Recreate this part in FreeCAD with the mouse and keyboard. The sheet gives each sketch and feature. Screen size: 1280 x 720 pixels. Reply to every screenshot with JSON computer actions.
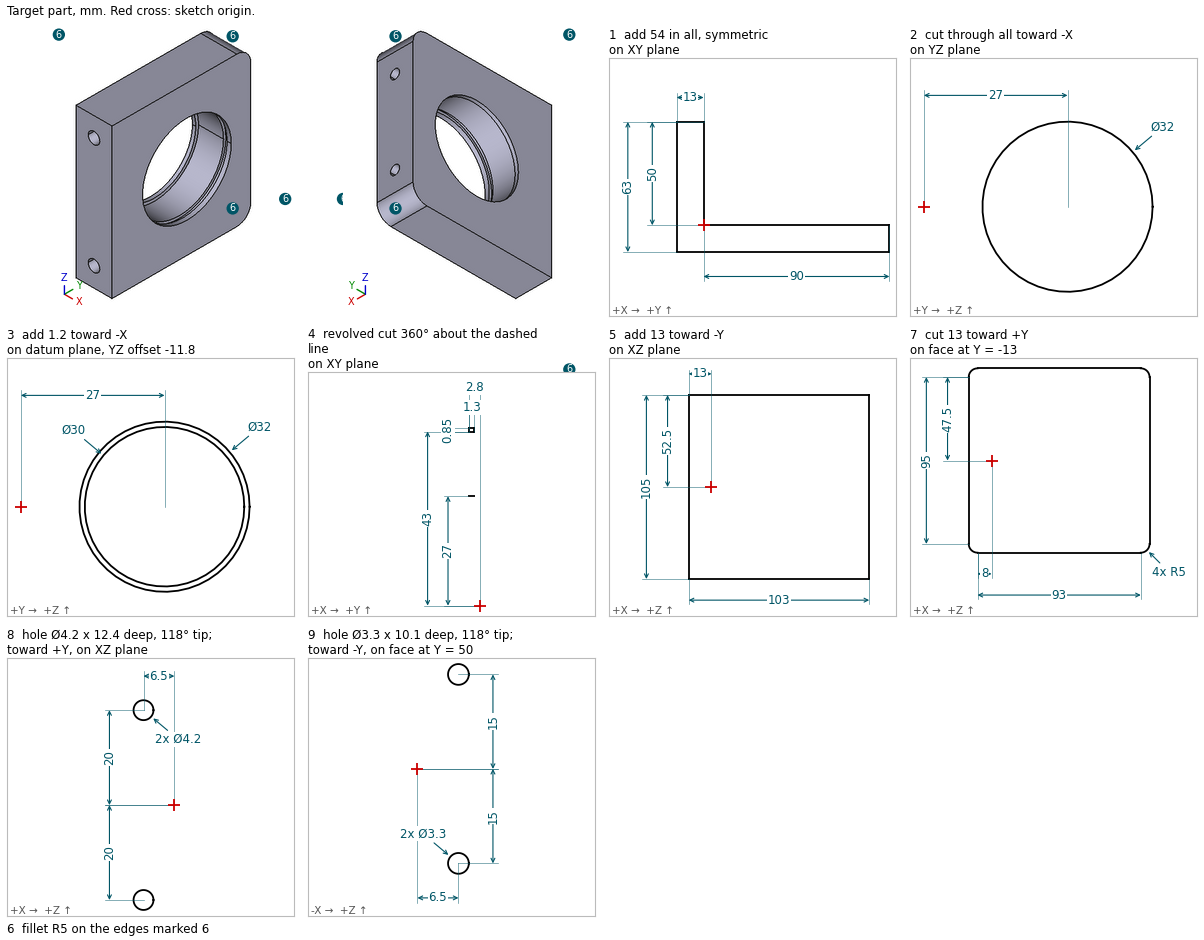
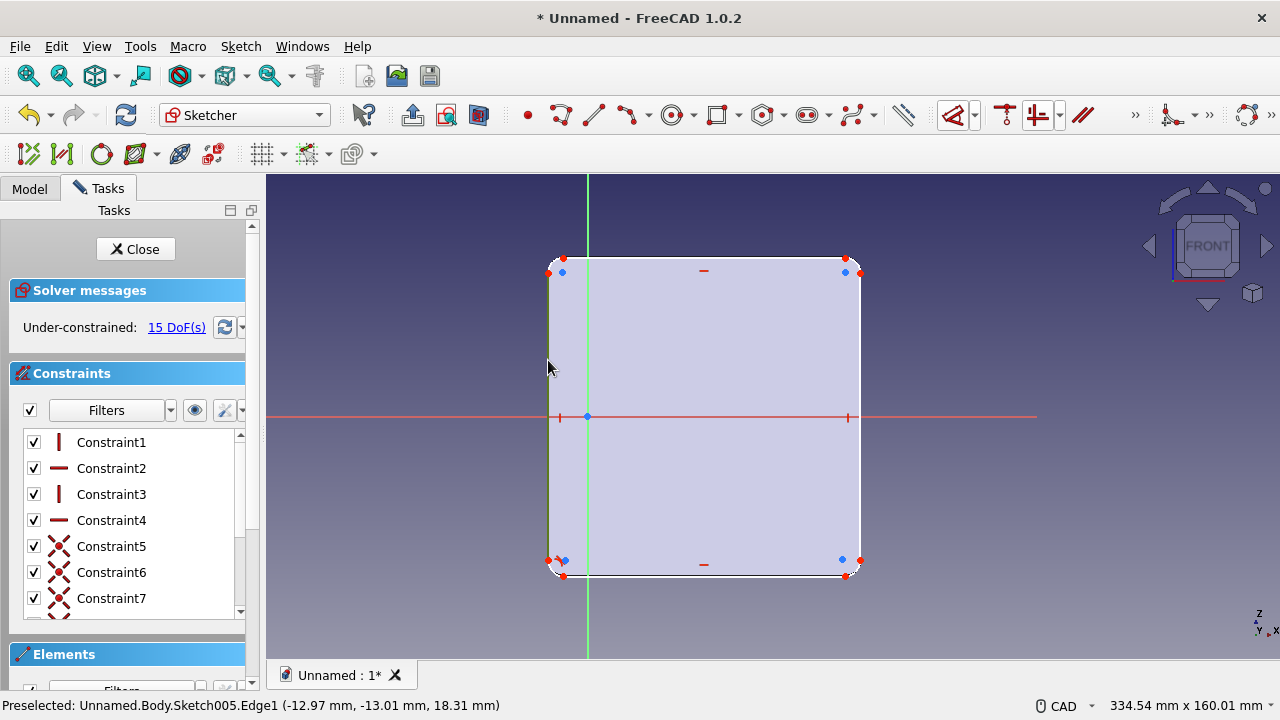
{"action": "left_click", "coordinate": [552, 263]}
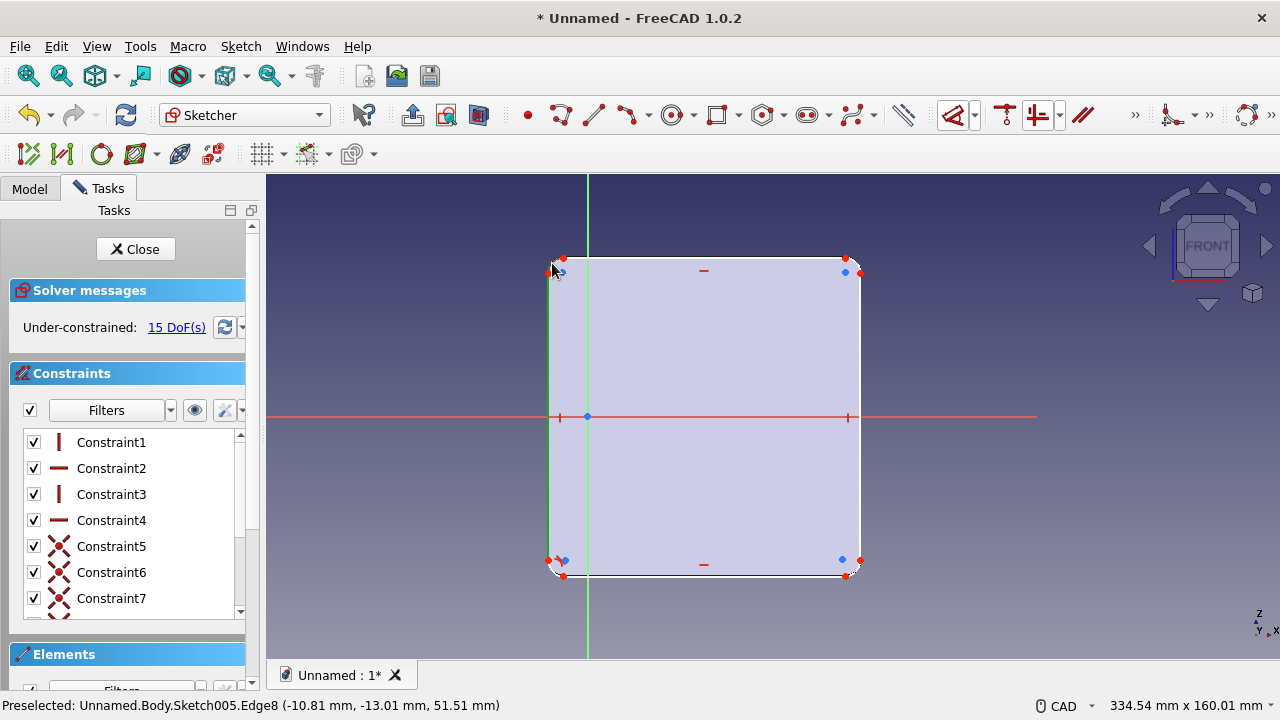
{"action": "key", "text": "t"}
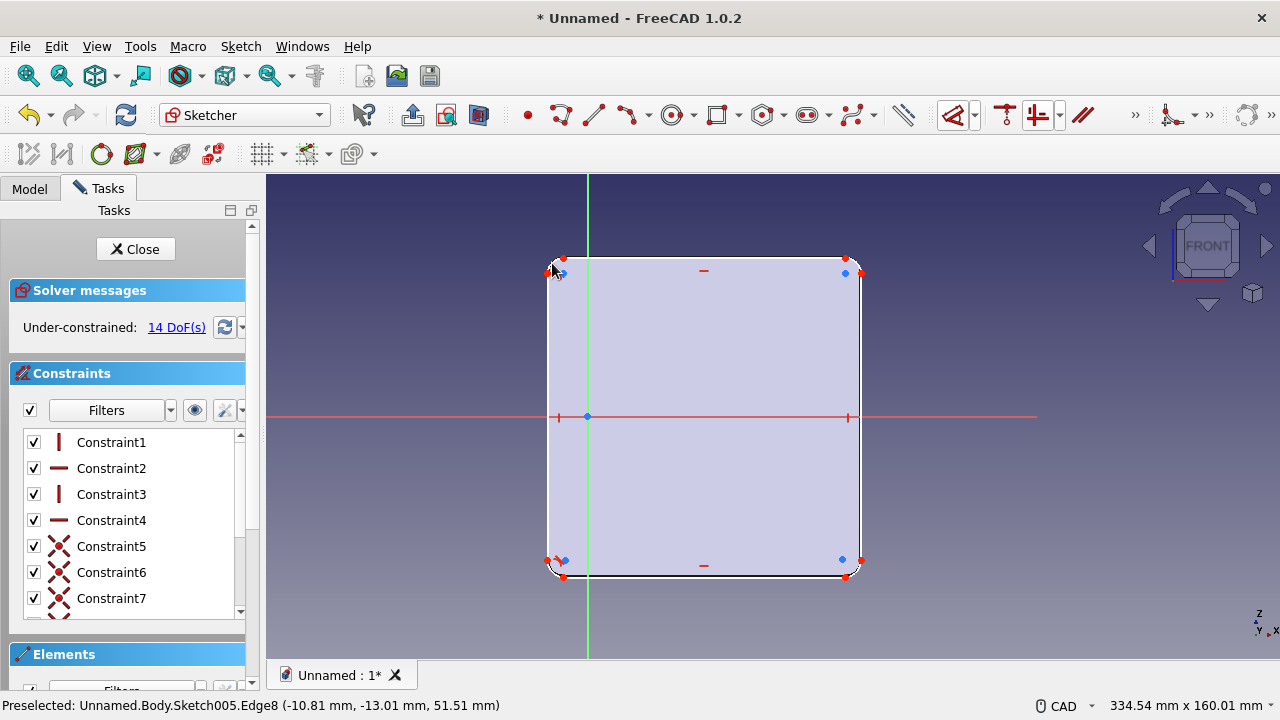
{"action": "left_click", "coordinate": [648, 578]}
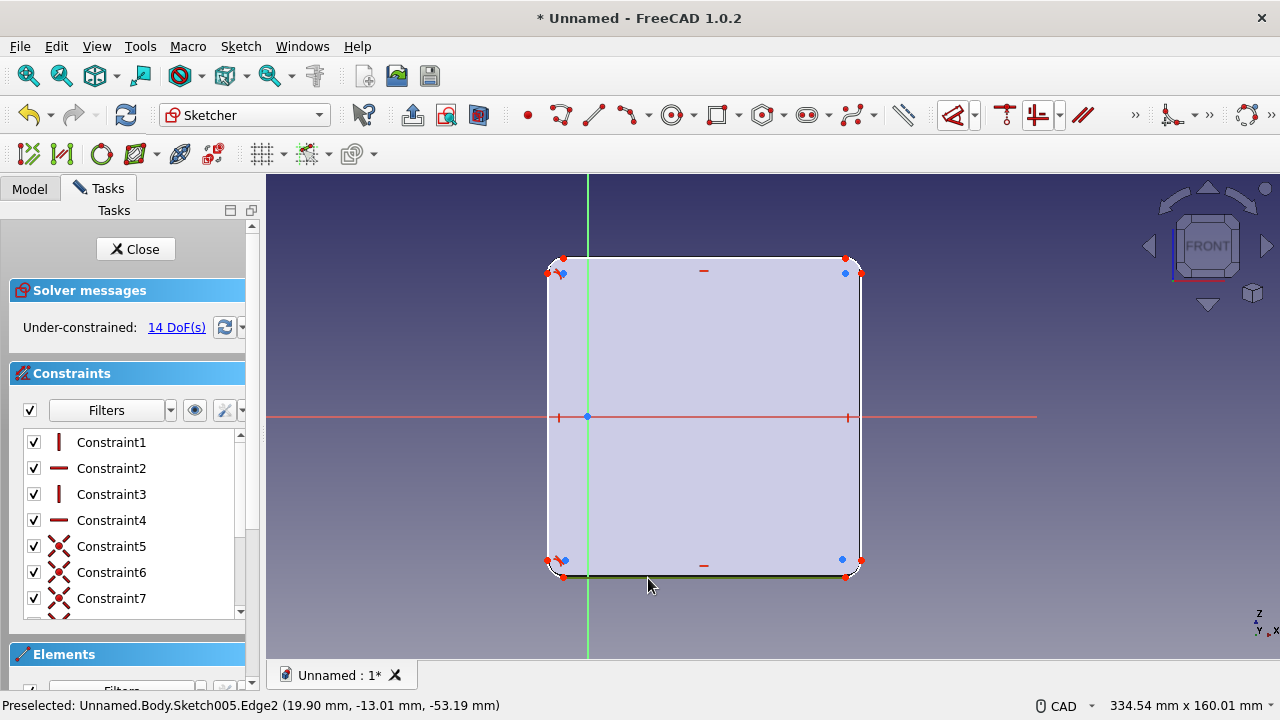
{"action": "left_click", "coordinate": [552, 572]}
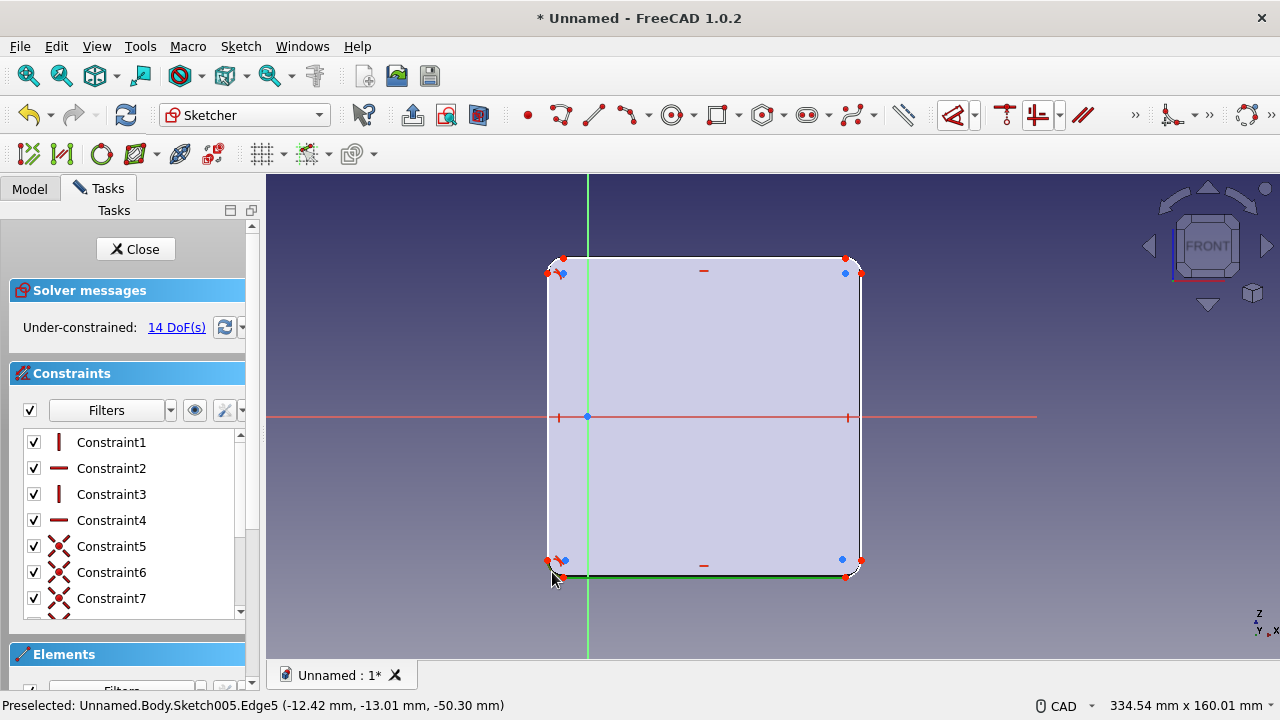
{"action": "key", "text": "t"}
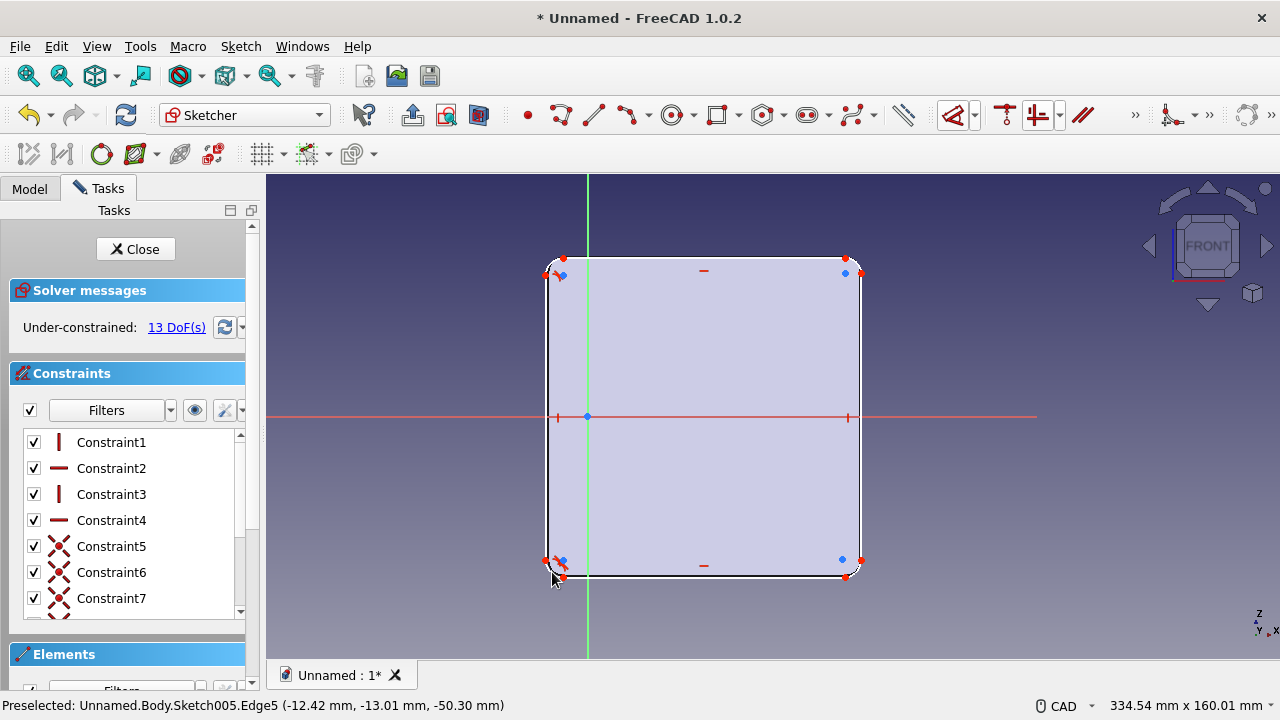
{"action": "left_click", "coordinate": [648, 578]}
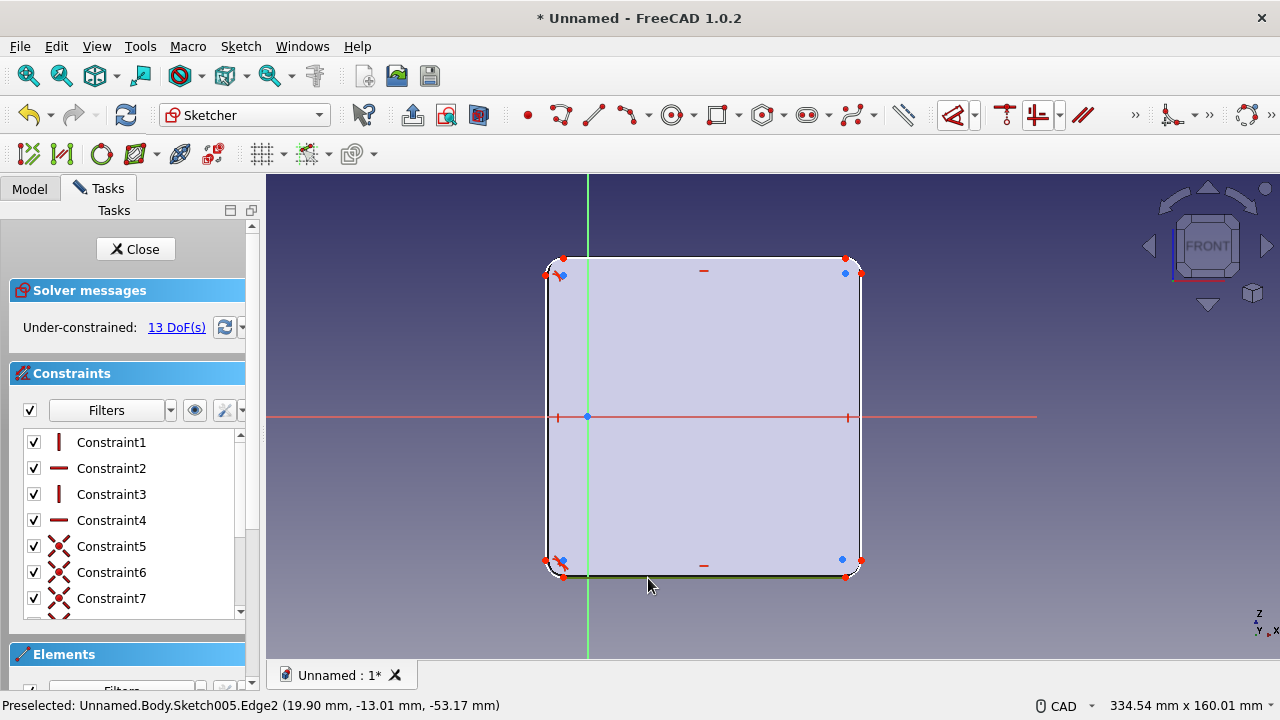
{"action": "left_click", "coordinate": [856, 572]}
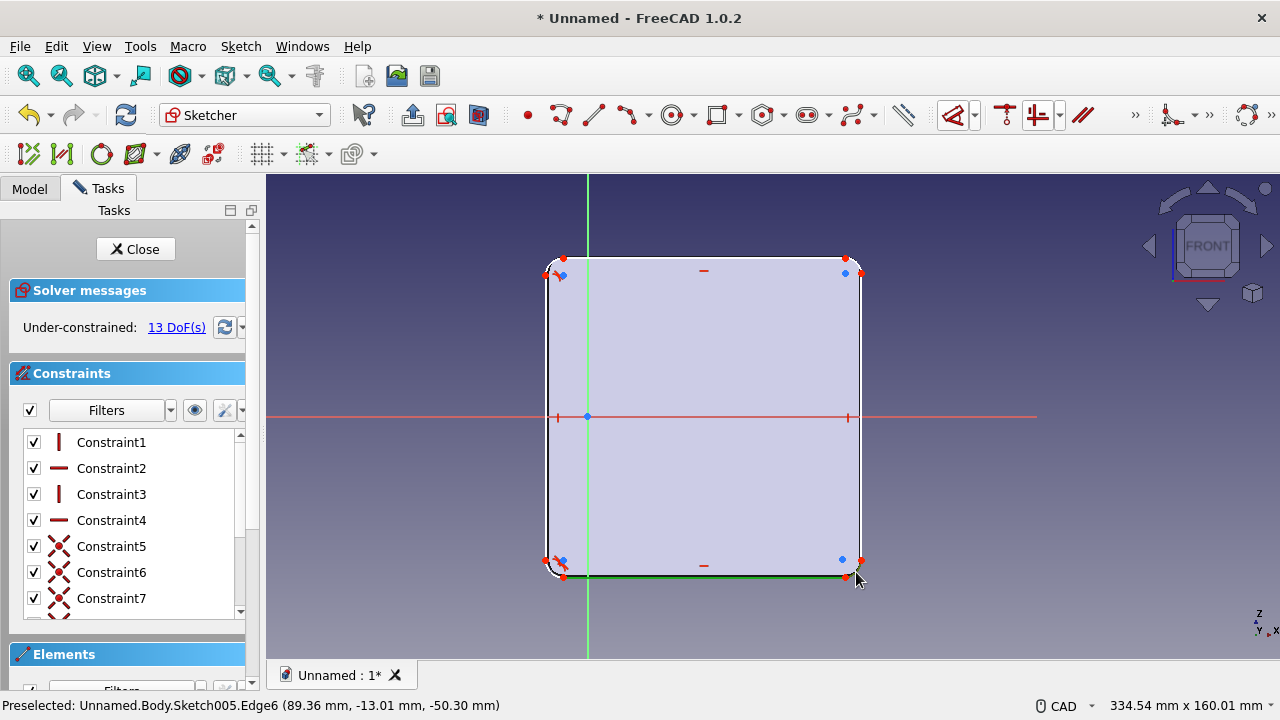
{"action": "key", "text": "t"}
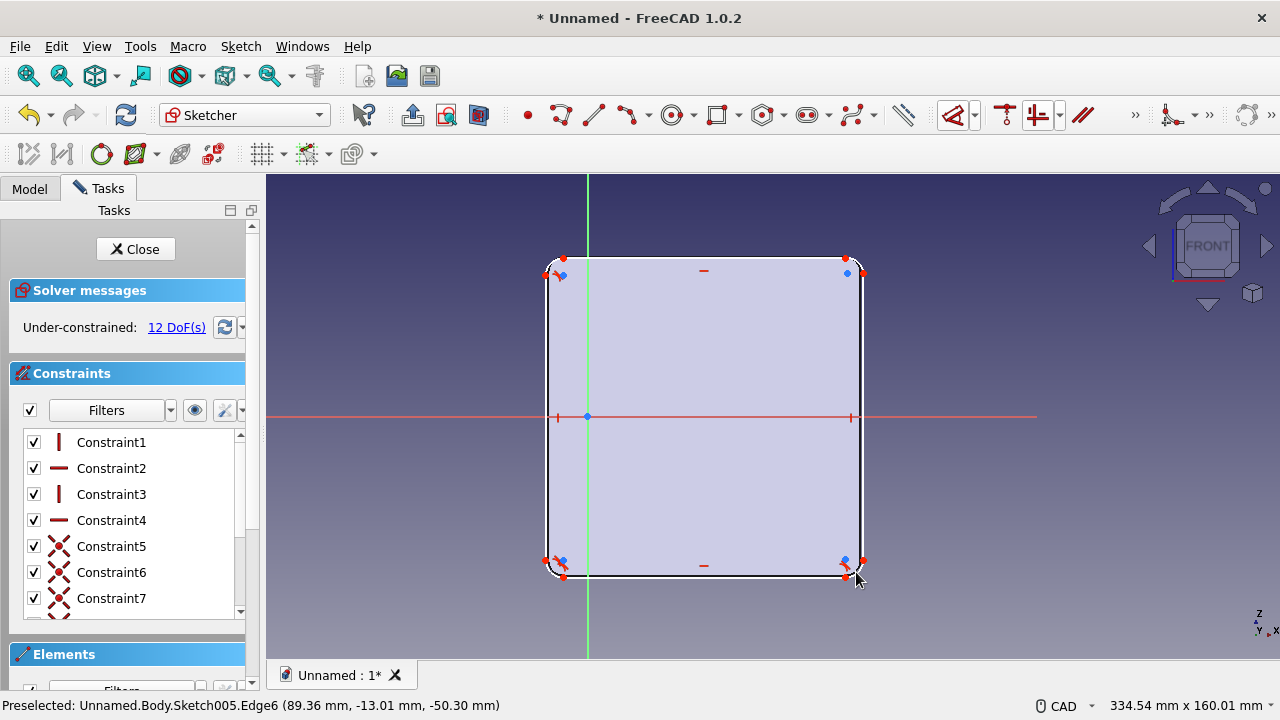
{"action": "left_click", "coordinate": [863, 475]}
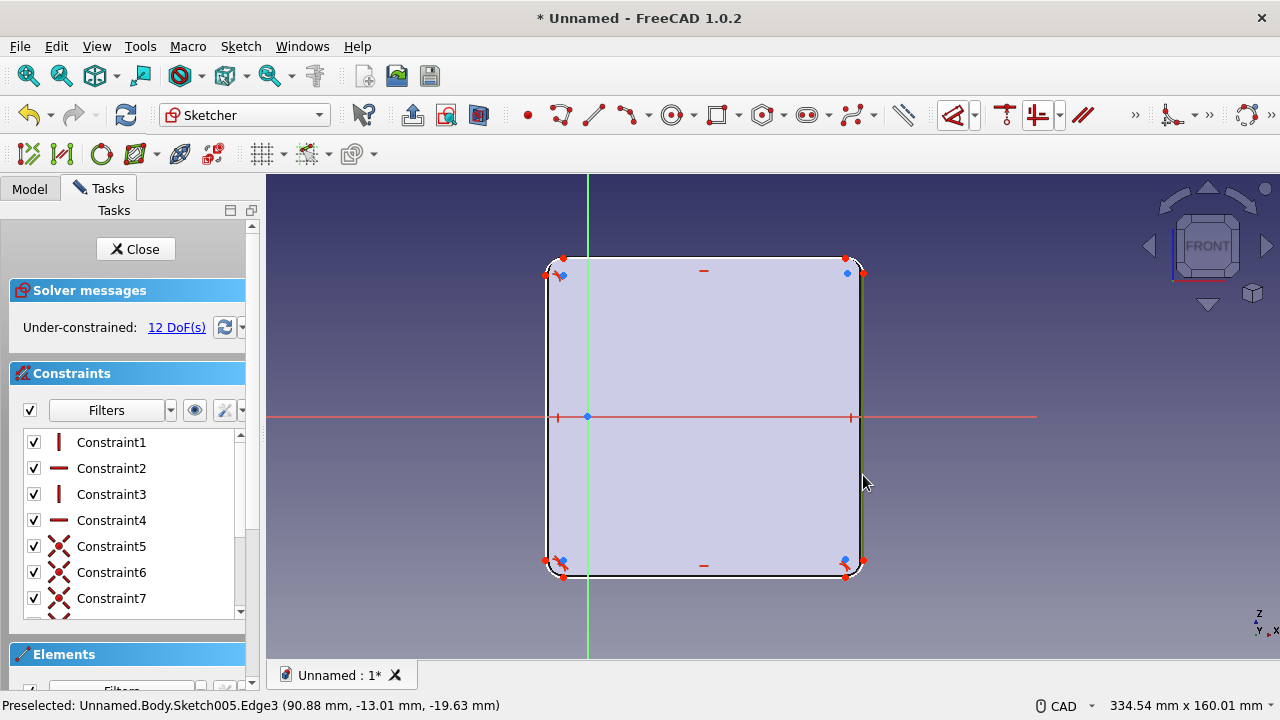
{"action": "left_click", "coordinate": [857, 573]}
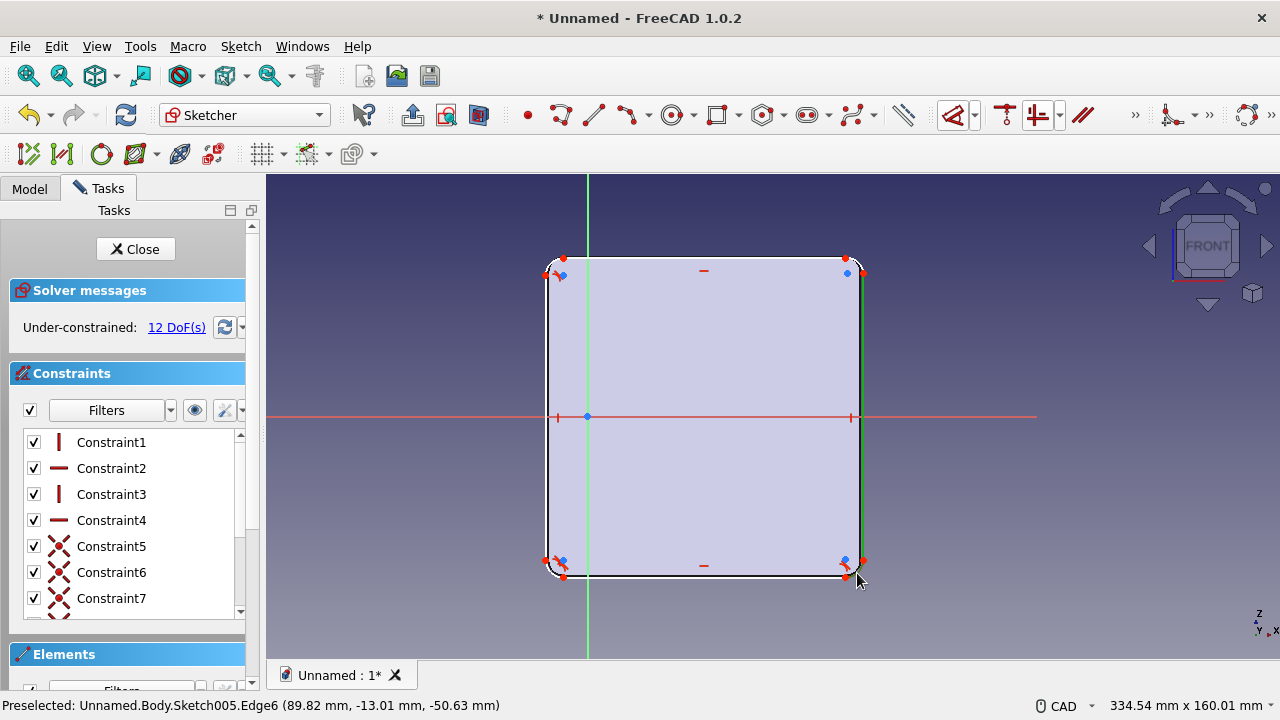
{"action": "key", "text": "t"}